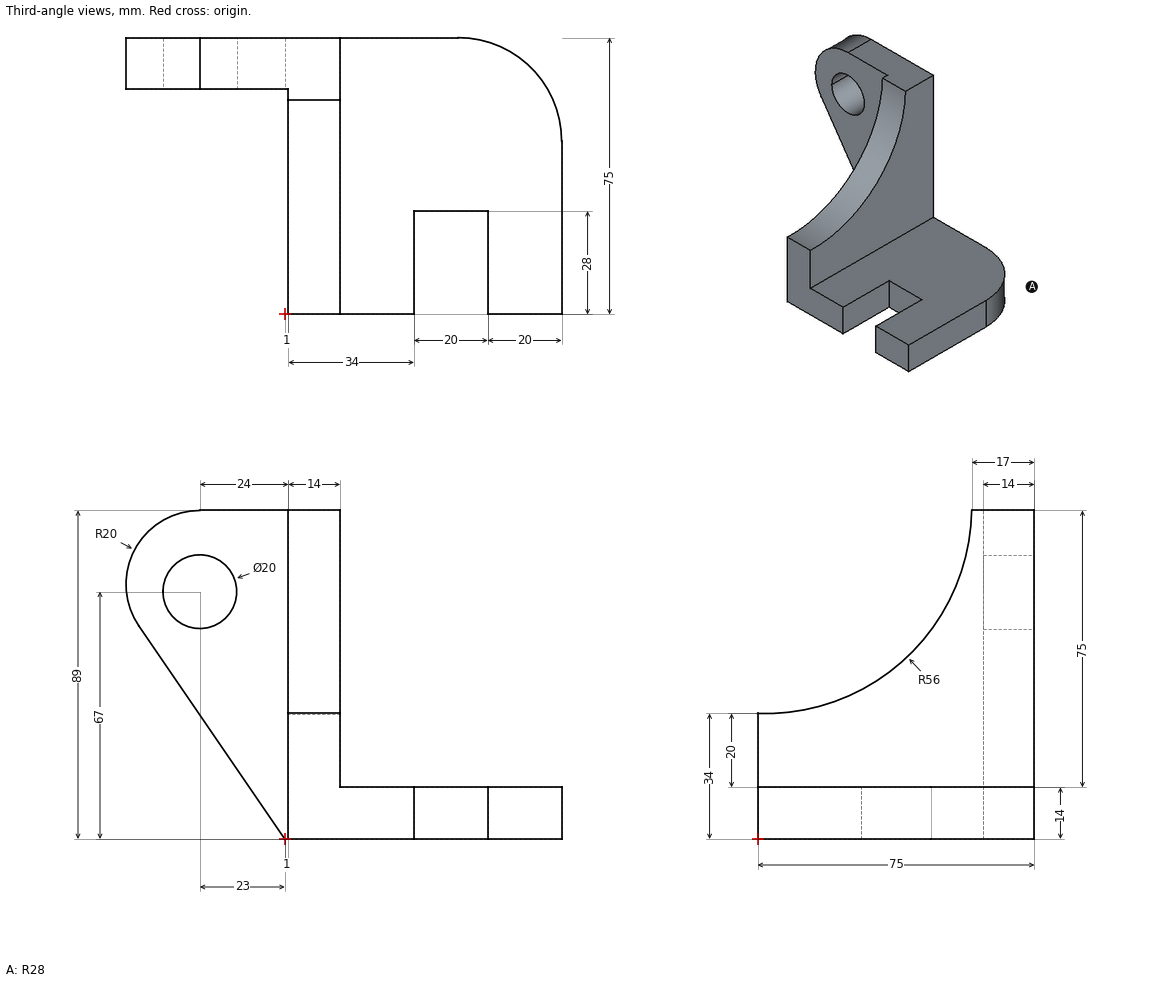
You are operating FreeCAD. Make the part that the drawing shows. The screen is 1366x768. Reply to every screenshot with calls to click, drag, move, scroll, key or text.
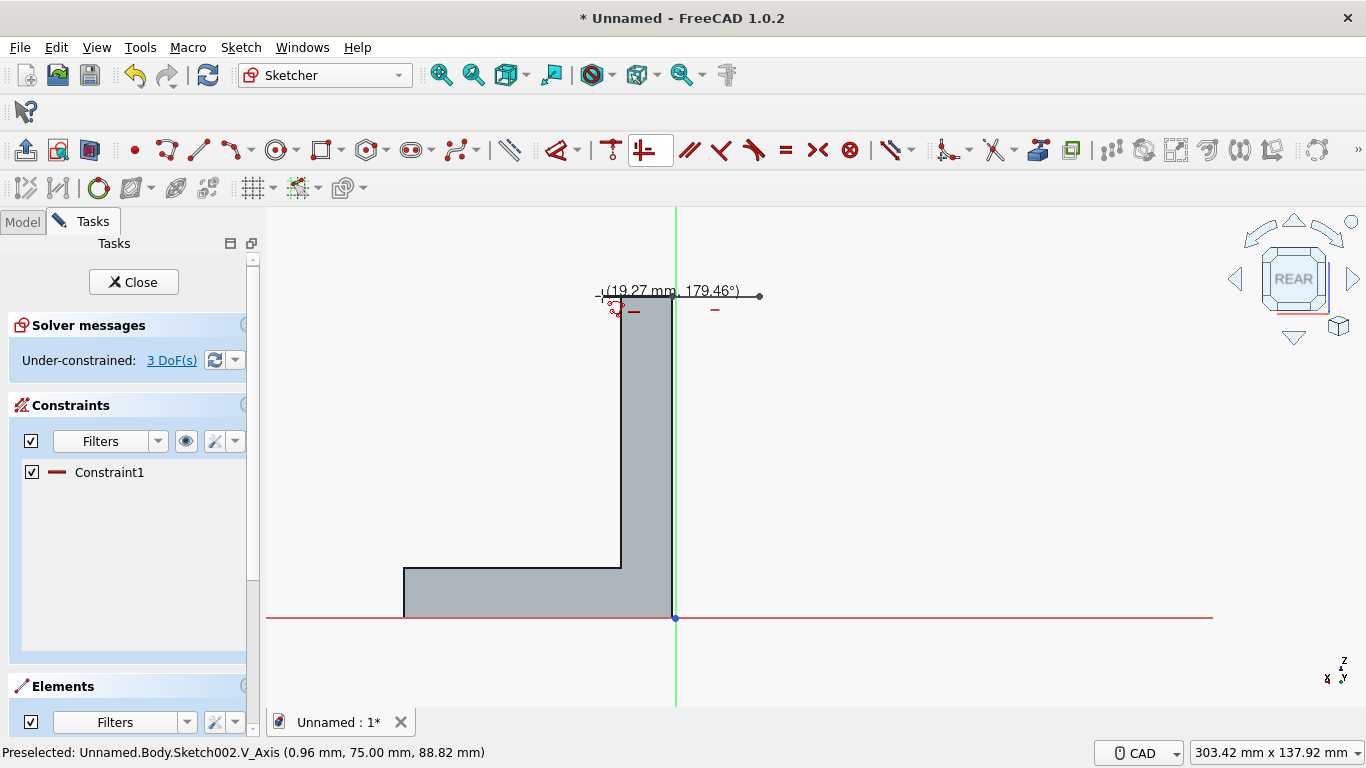
scroll(672, 618, up, 8)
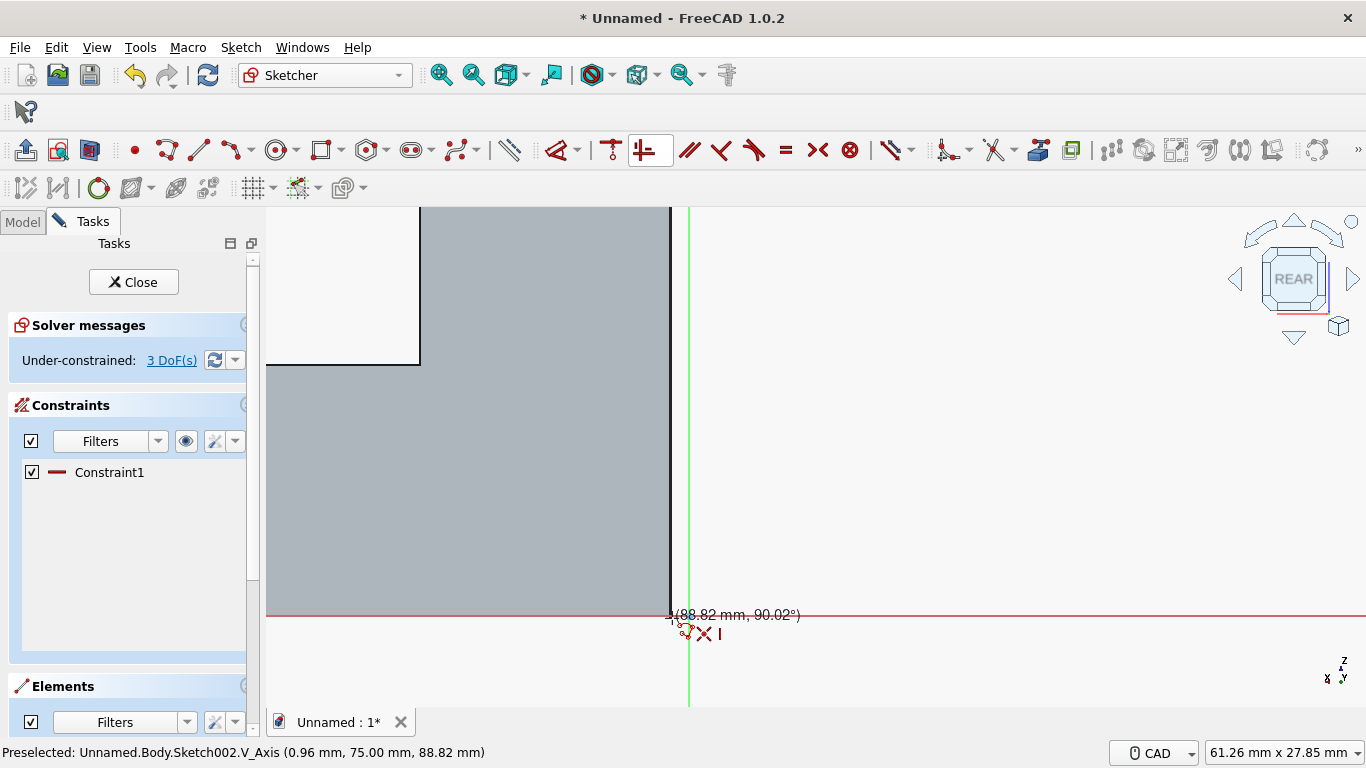
click(671, 616)
click(689, 616)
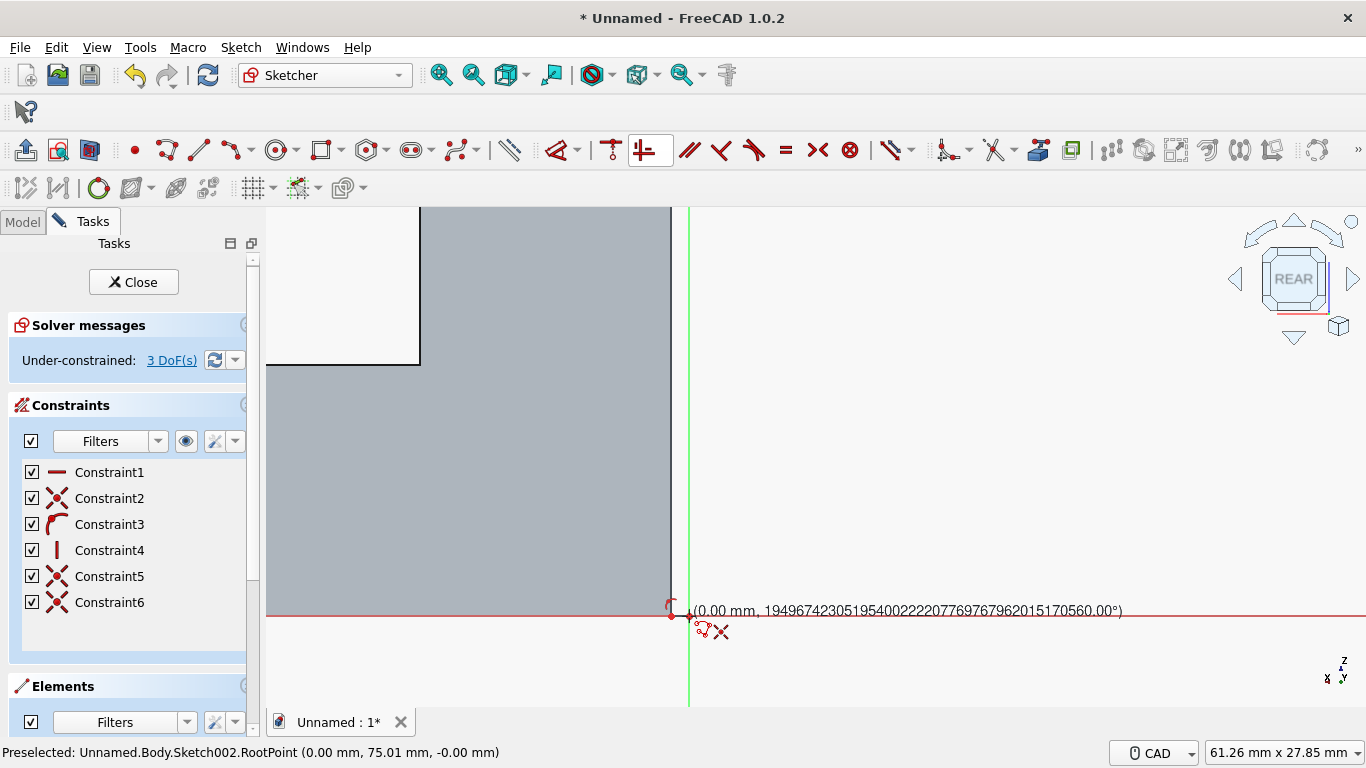
scroll(672, 619, down, 8)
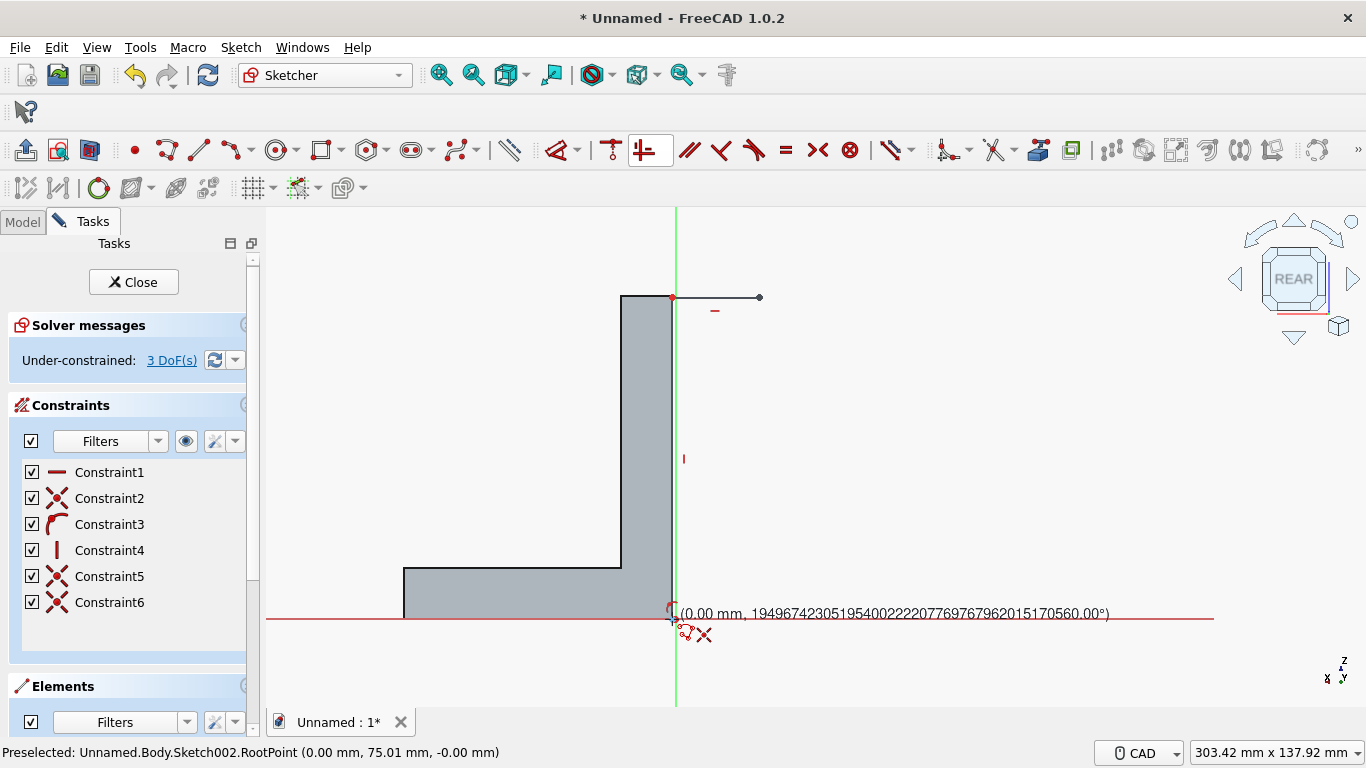
click(819, 410)
right_click(819, 410)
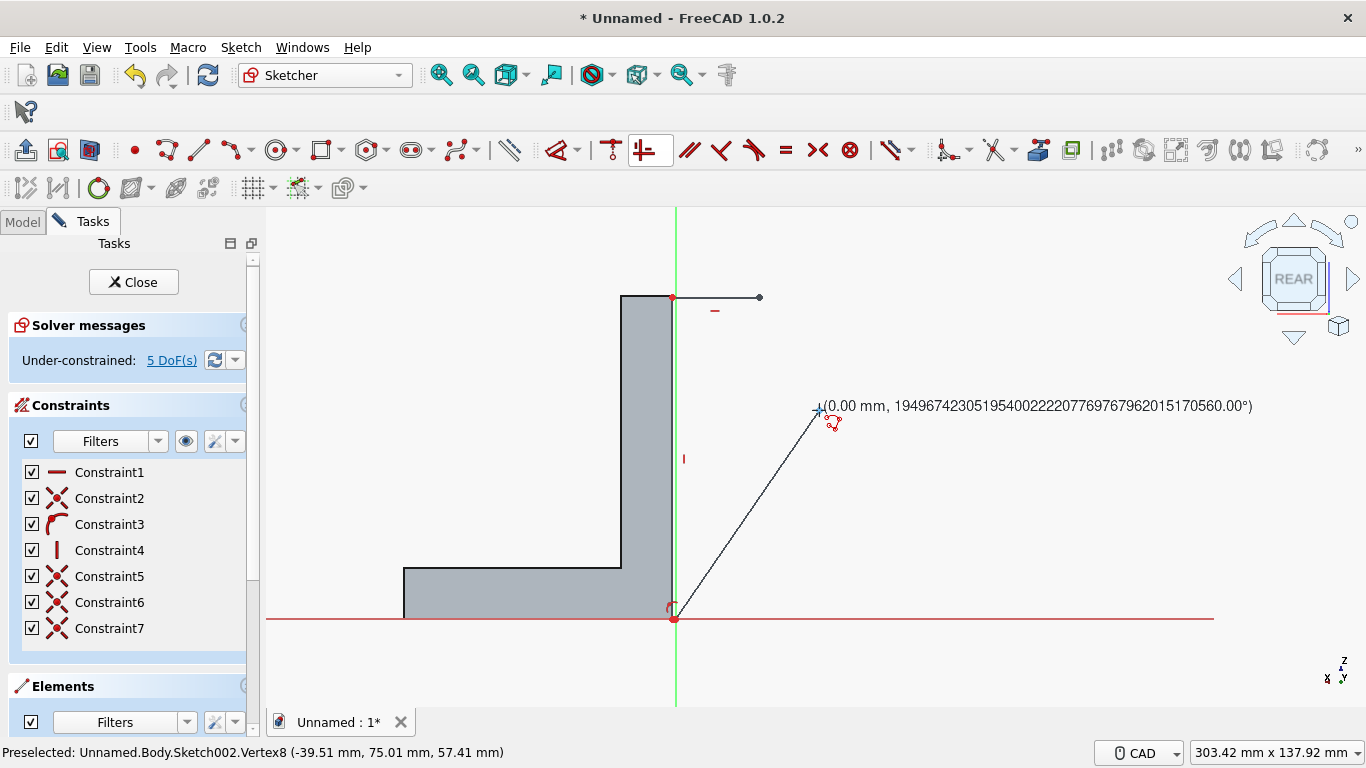
click(232, 150)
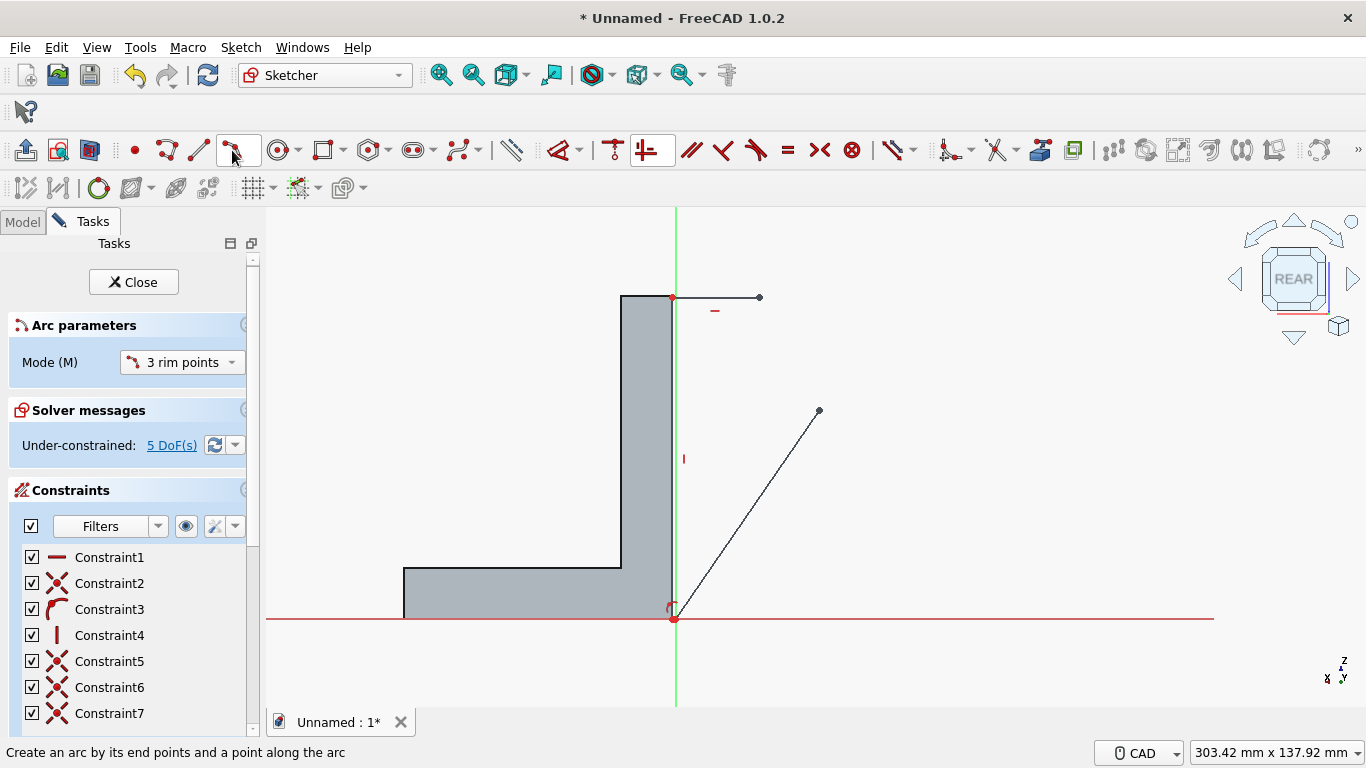
click(819, 411)
click(759, 298)
click(823, 335)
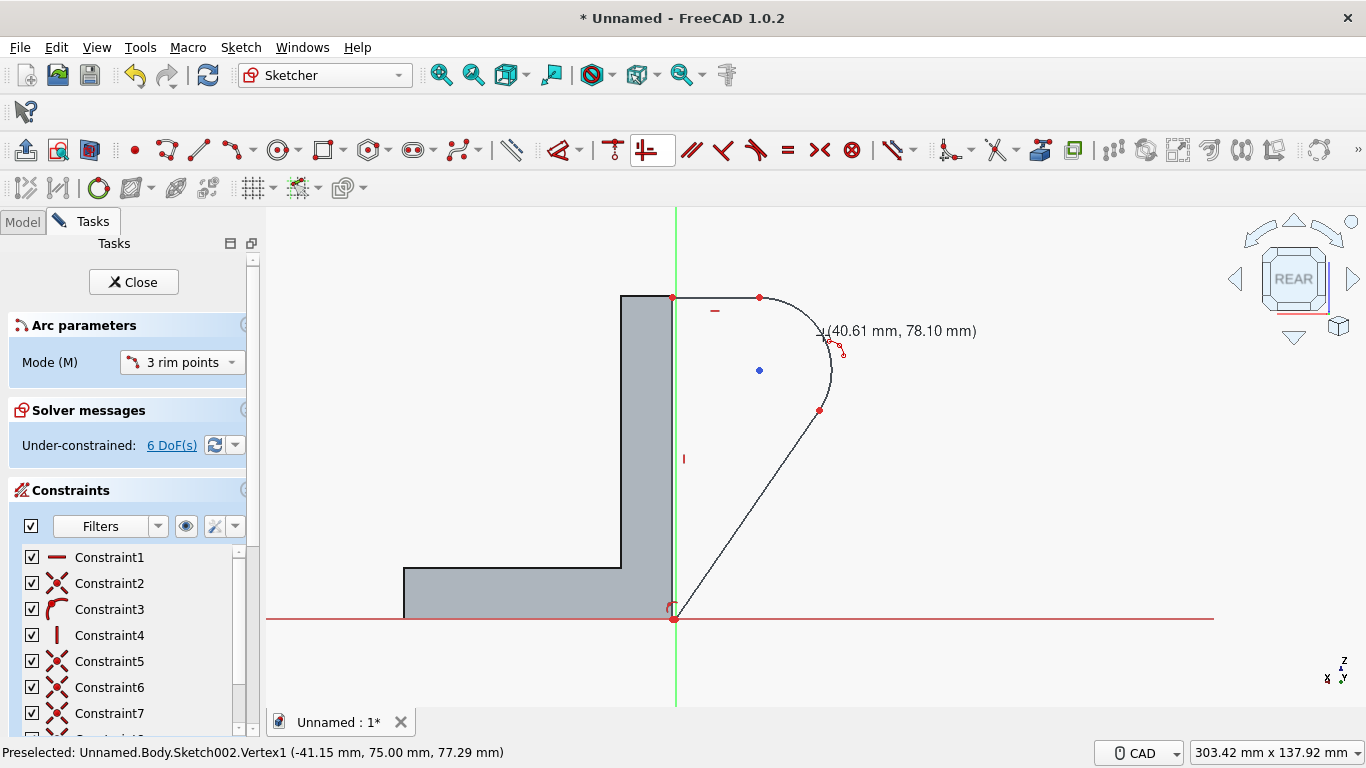
click(278, 150)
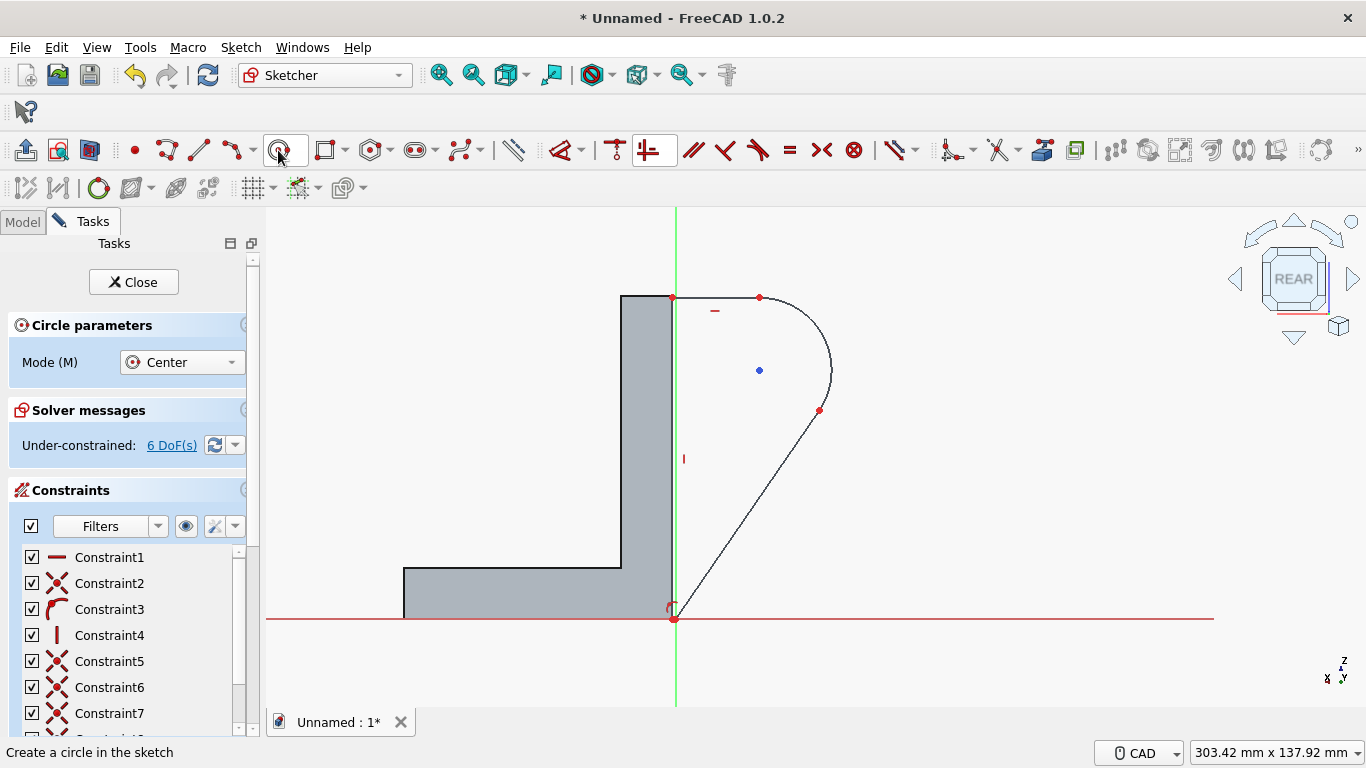
scroll(759, 376, up, 4)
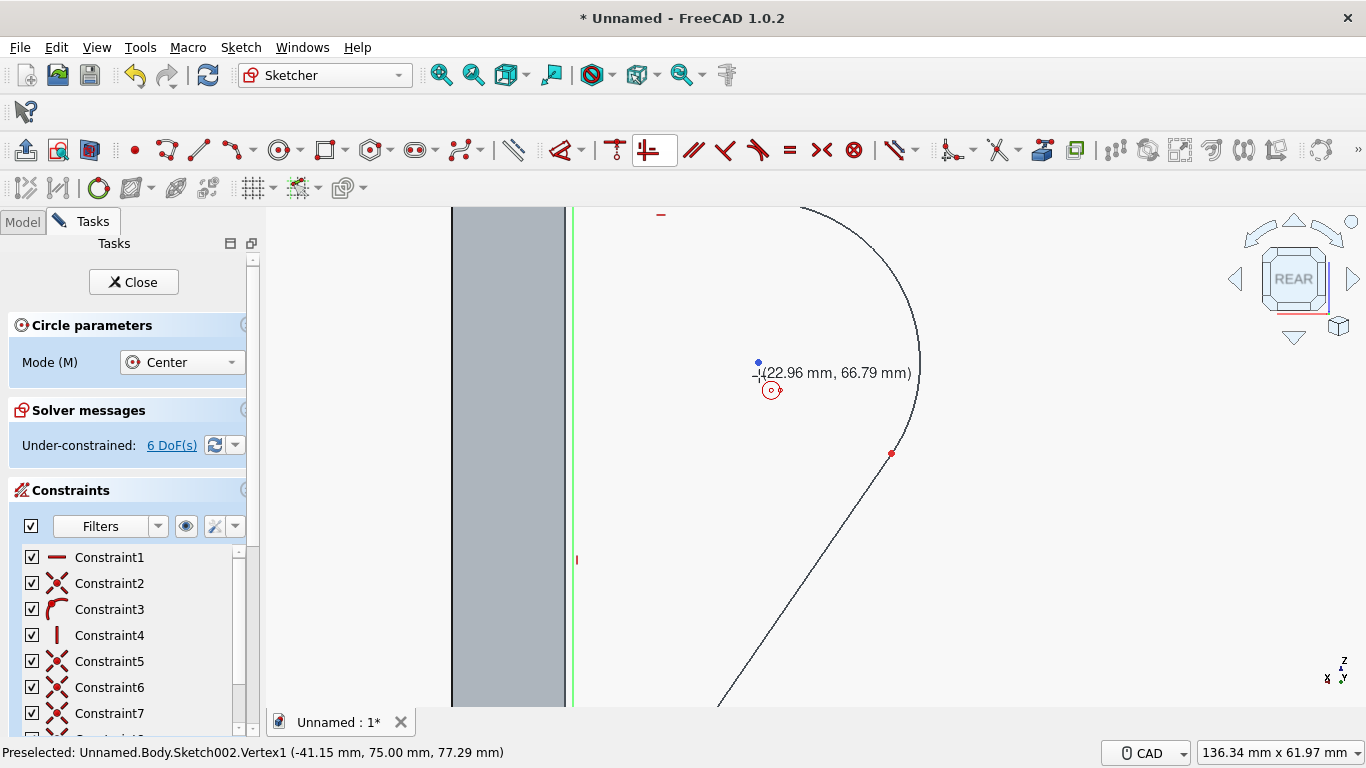
click(759, 376)
click(816, 319)
key(Escape)